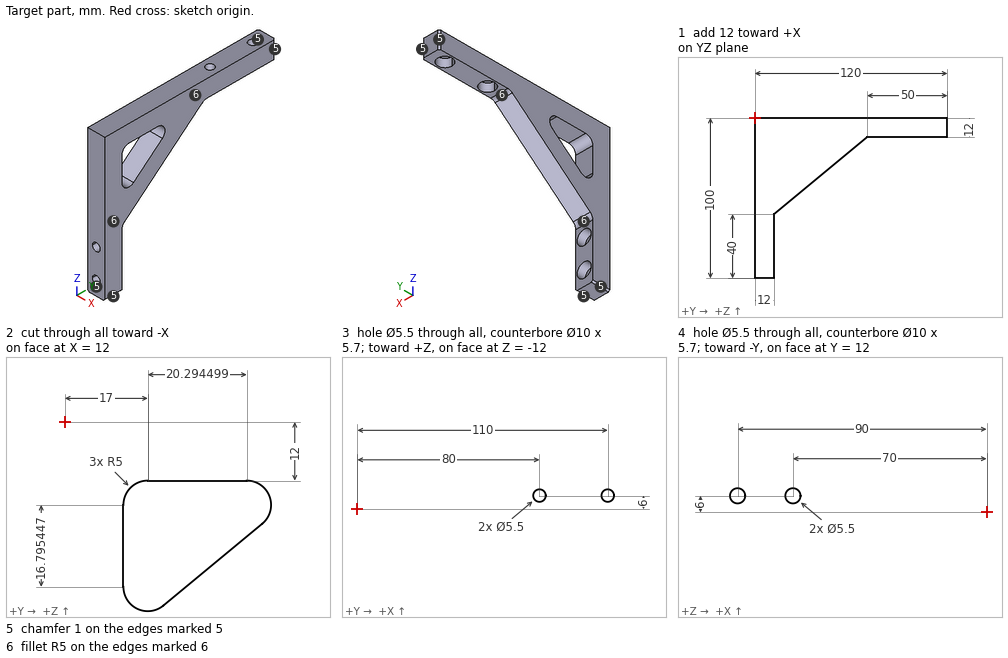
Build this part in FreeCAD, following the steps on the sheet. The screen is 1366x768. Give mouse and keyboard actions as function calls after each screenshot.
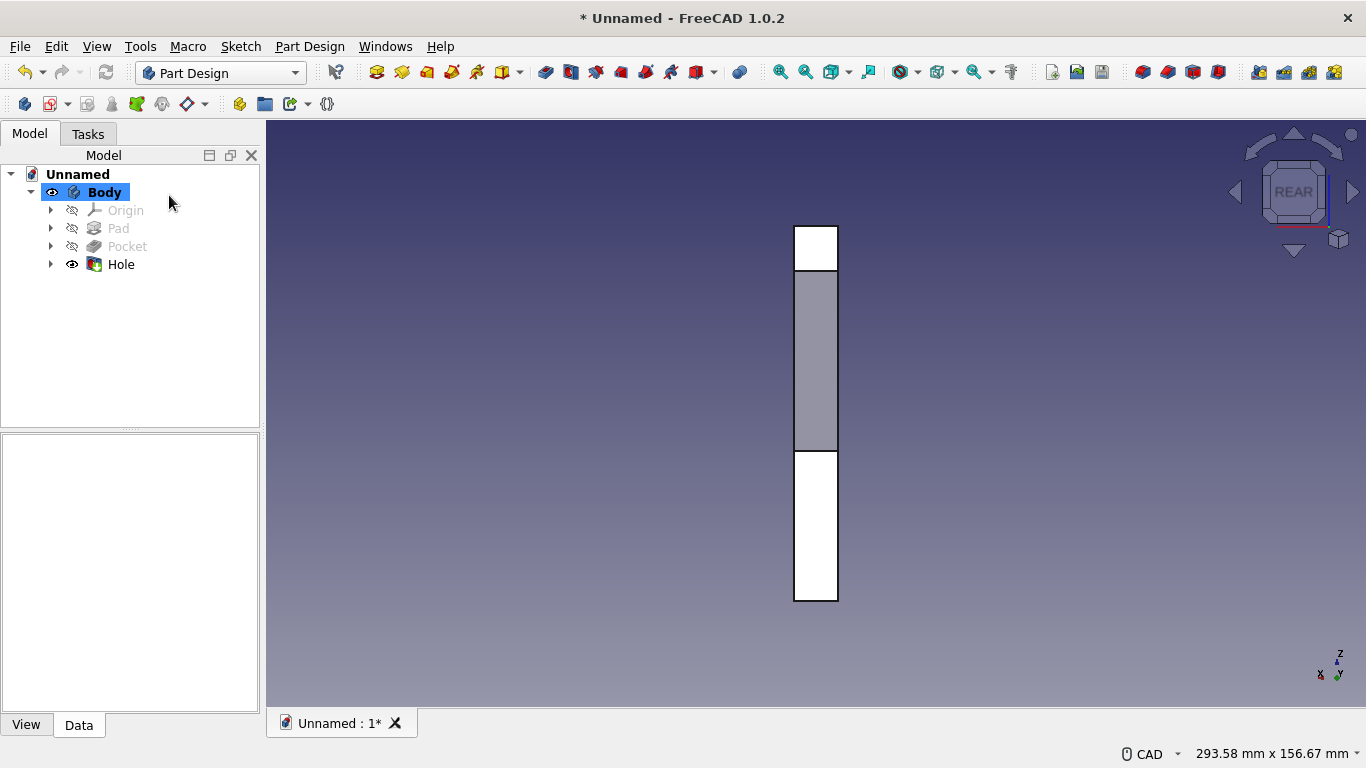
click(816, 546)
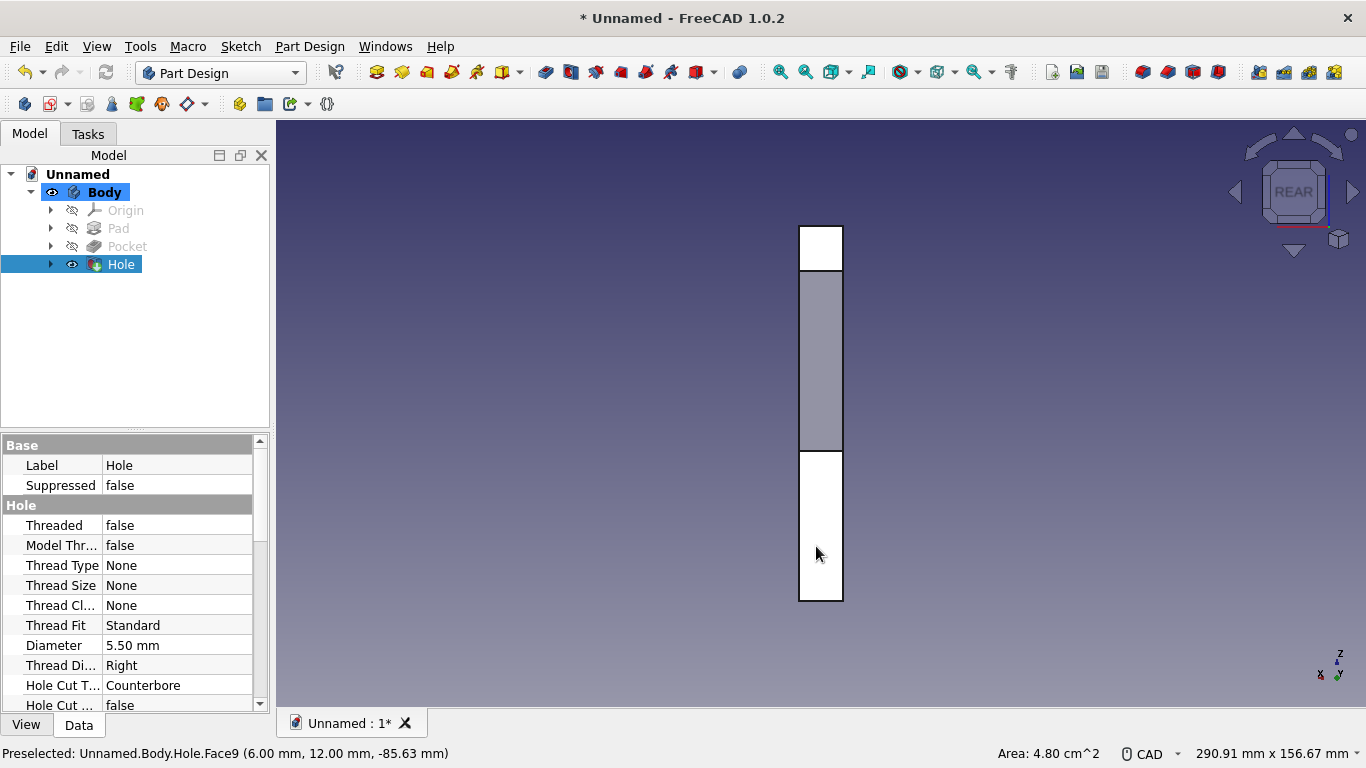
click(50, 104)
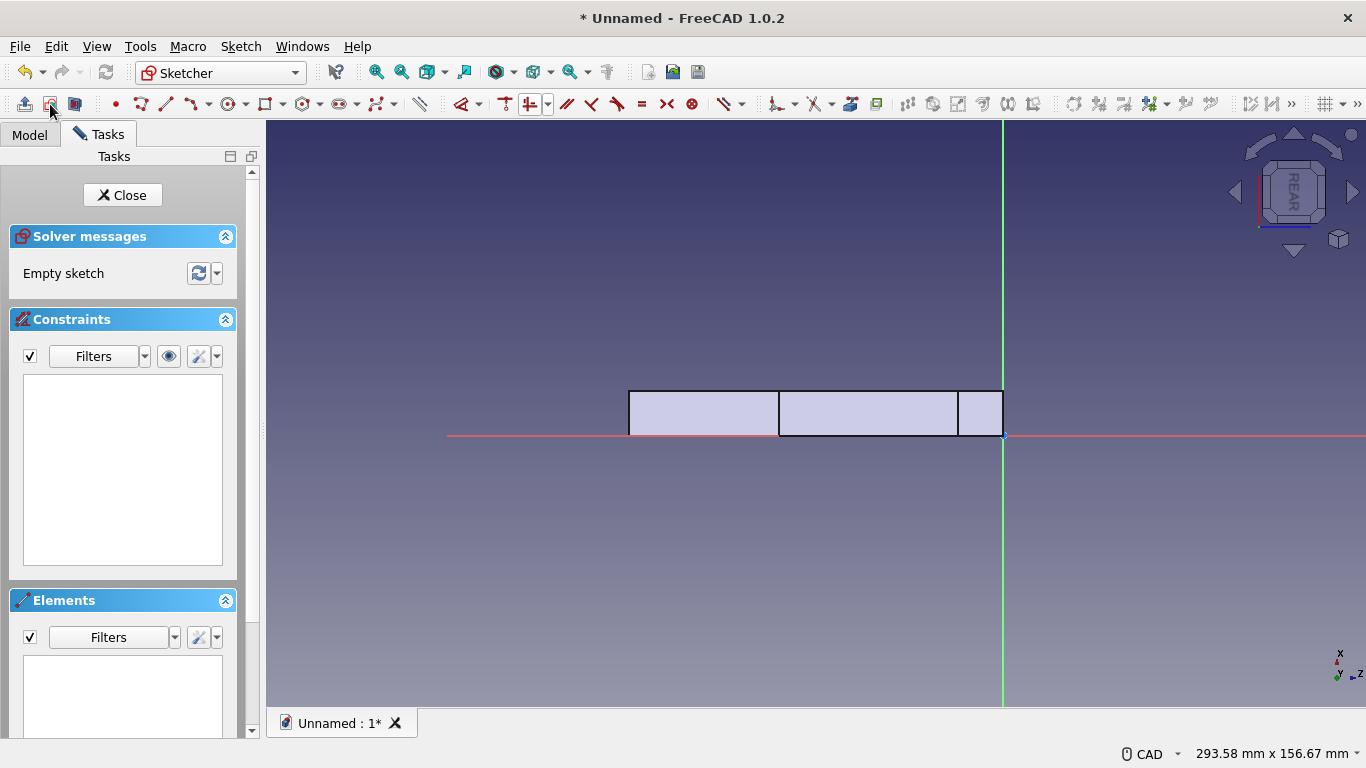
scroll(697, 414, up, 10)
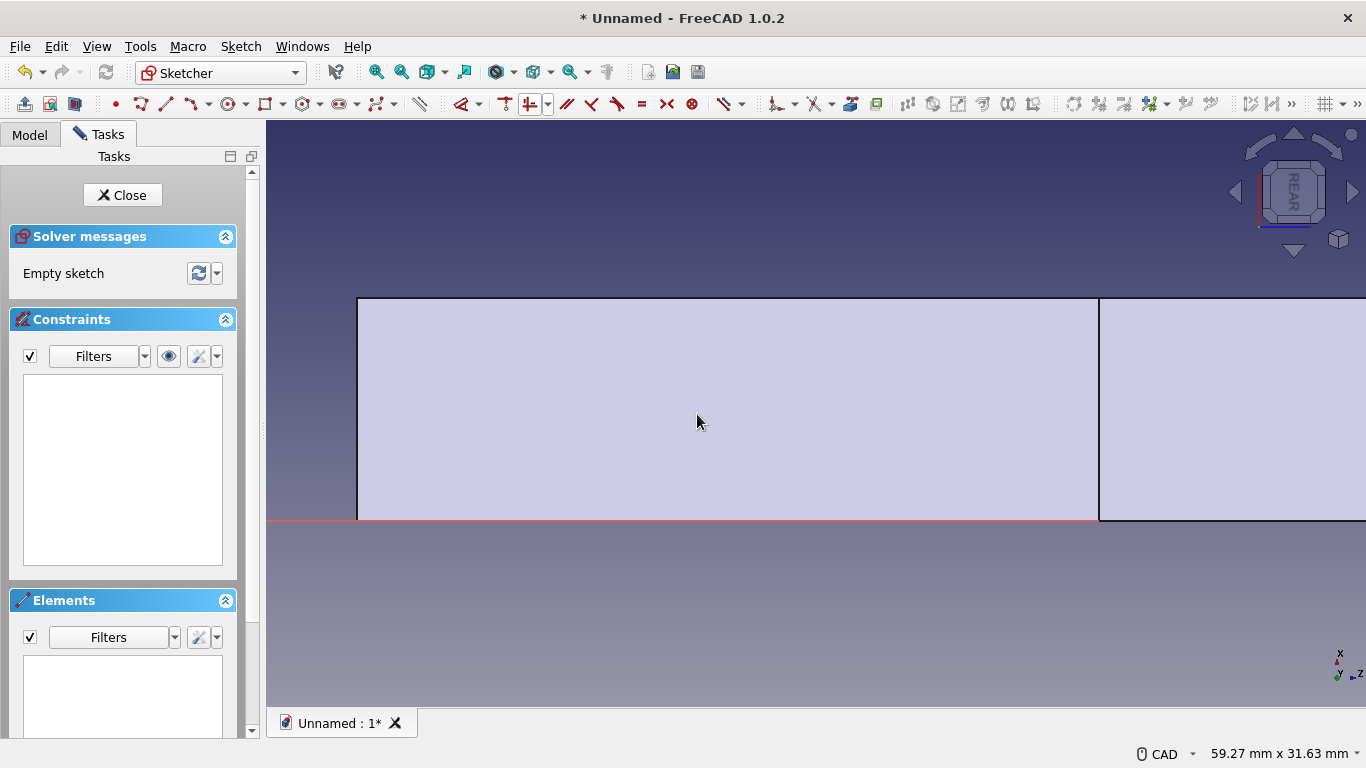
click(228, 104)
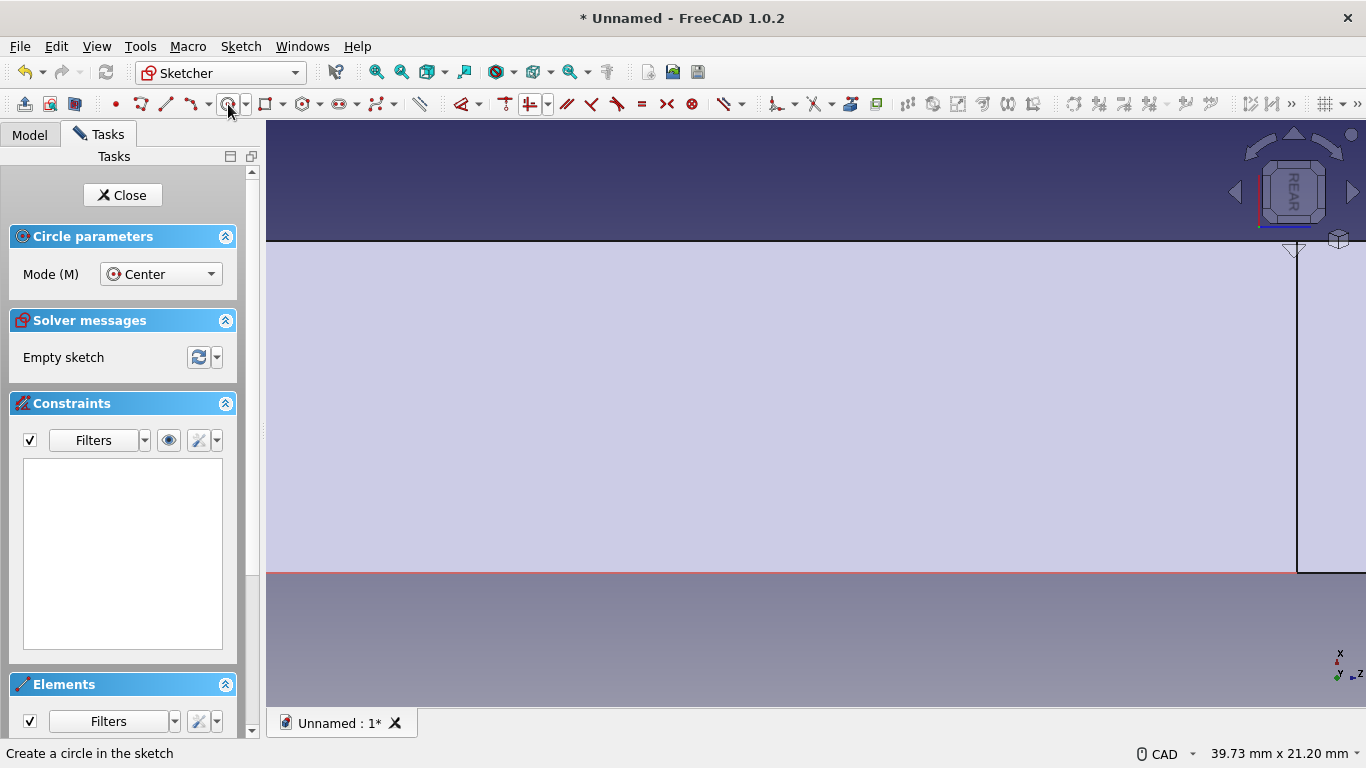
click(1020, 407)
click(1074, 353)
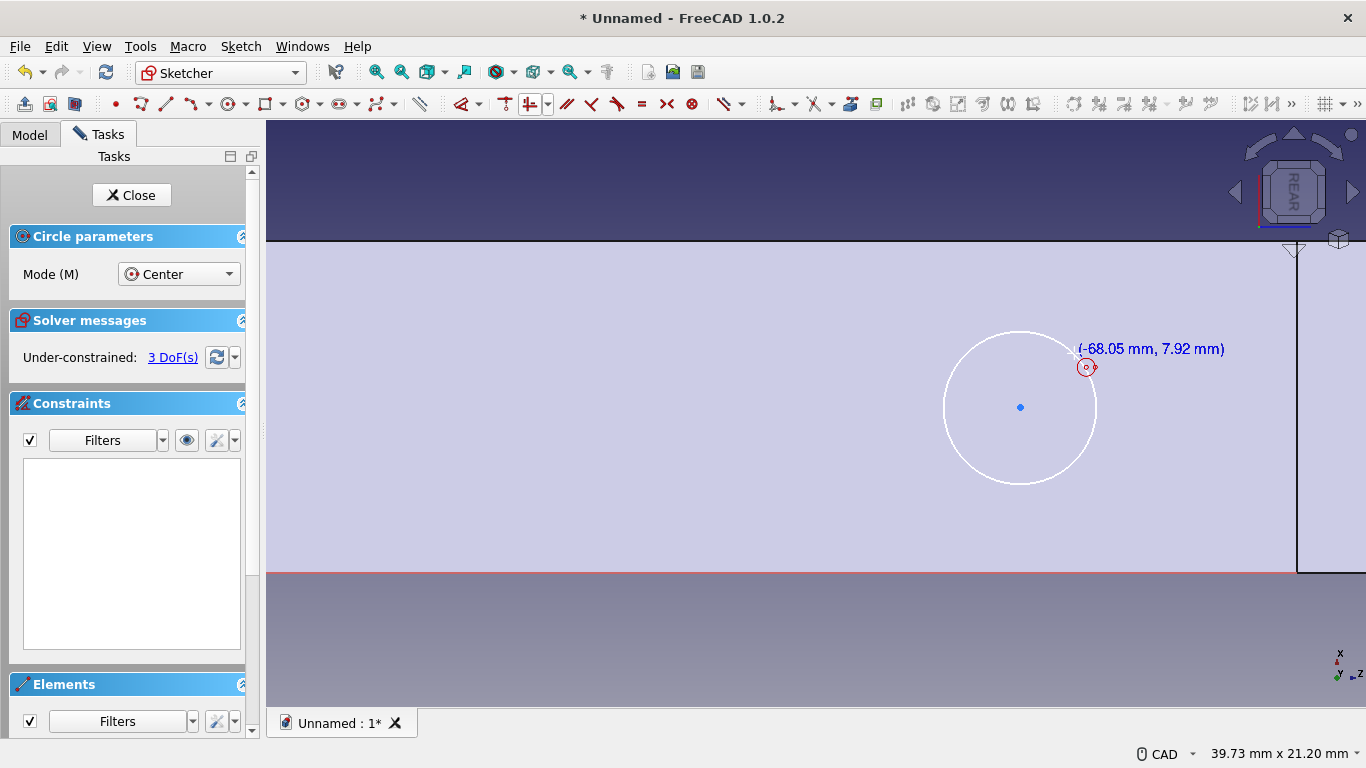
click(466, 407)
click(520, 353)
key(Escape)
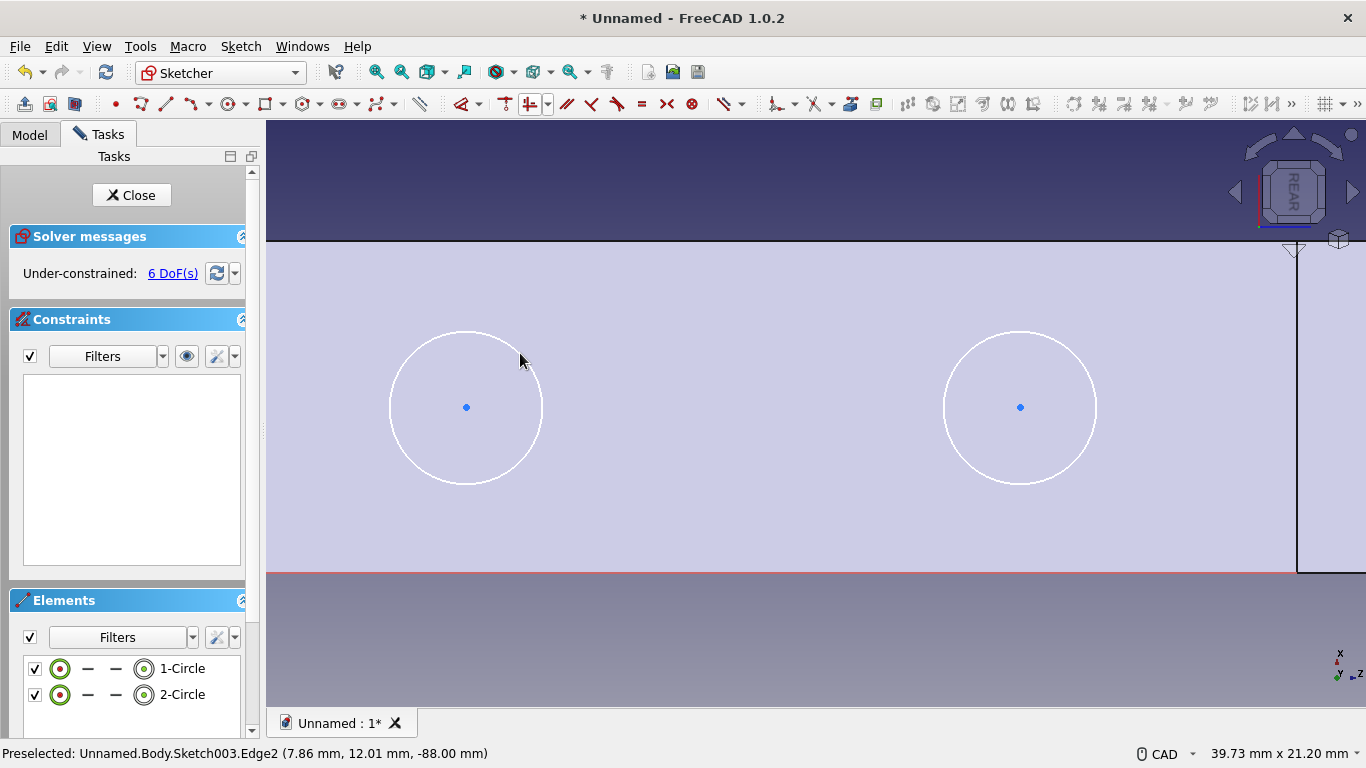
click(1074, 354)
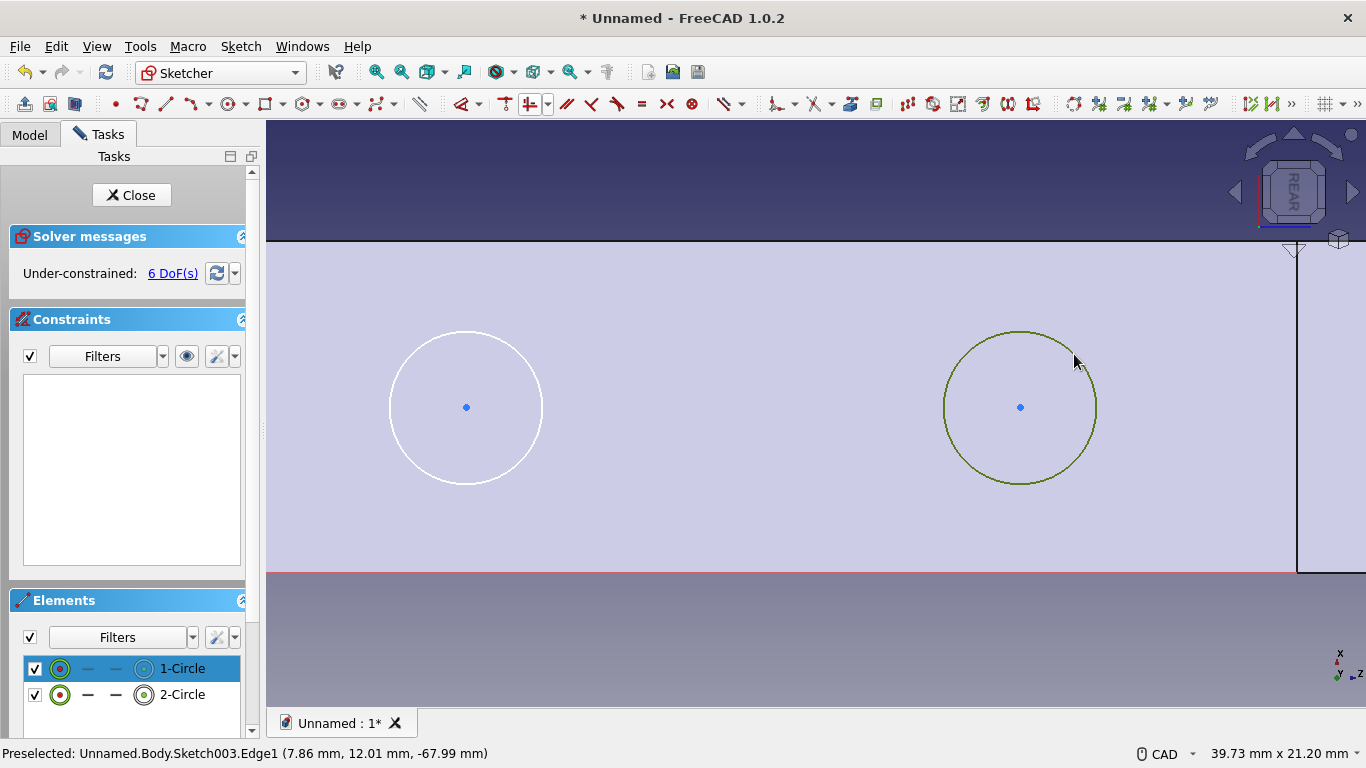
click(520, 354)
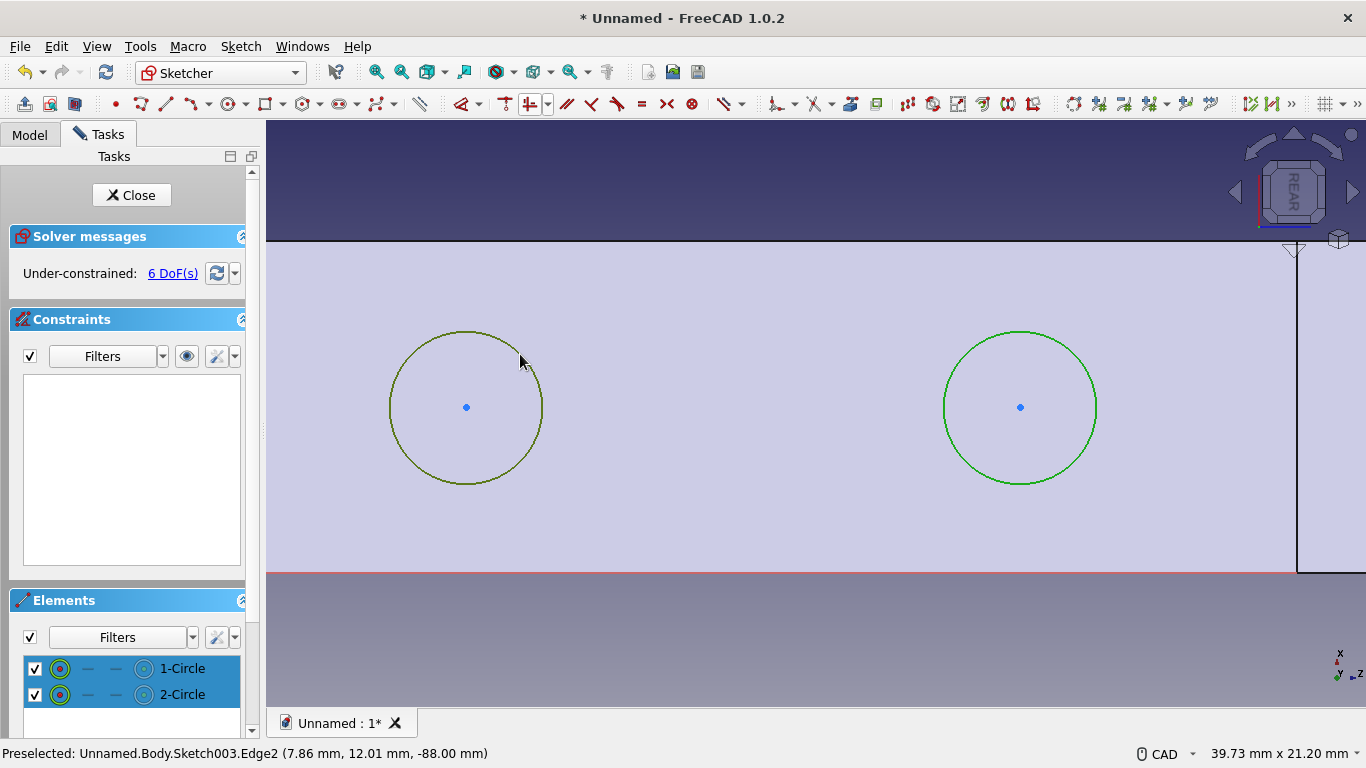
click(642, 104)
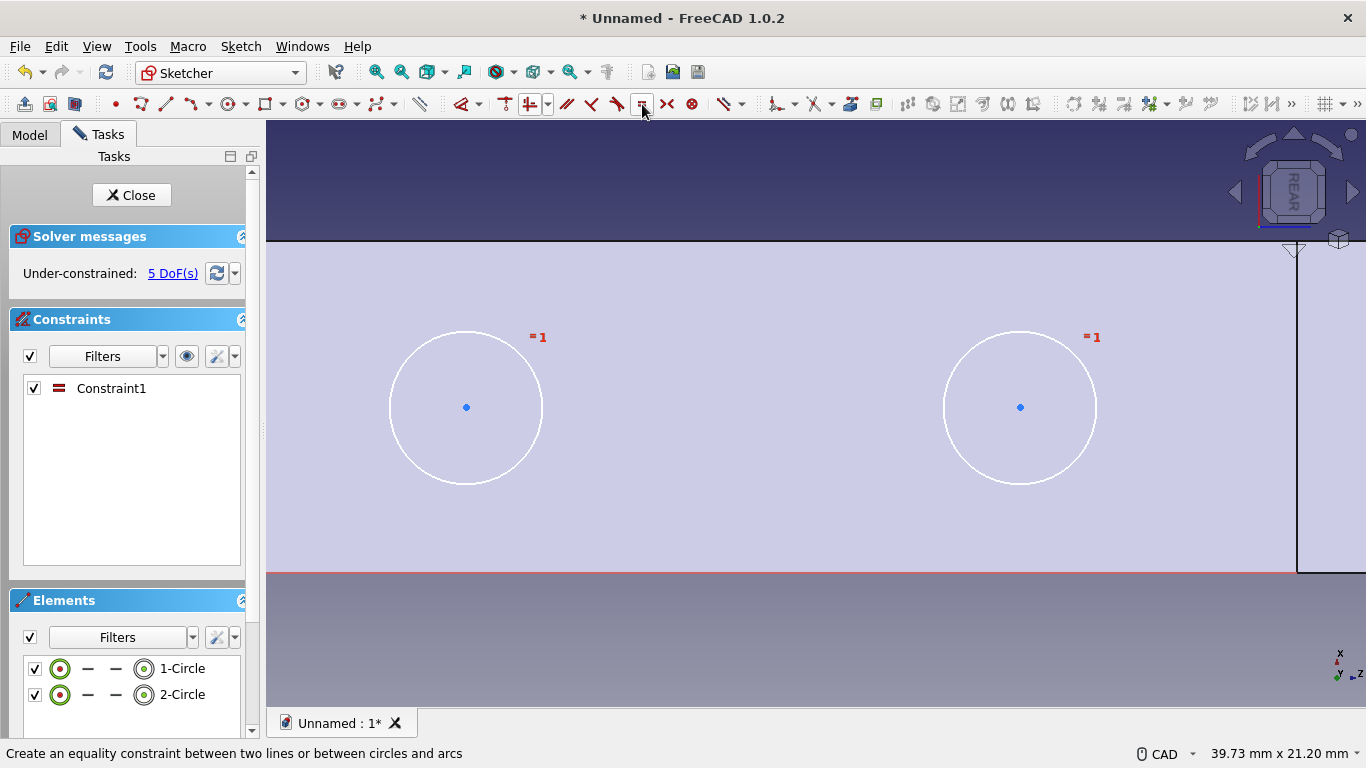
click(1020, 408)